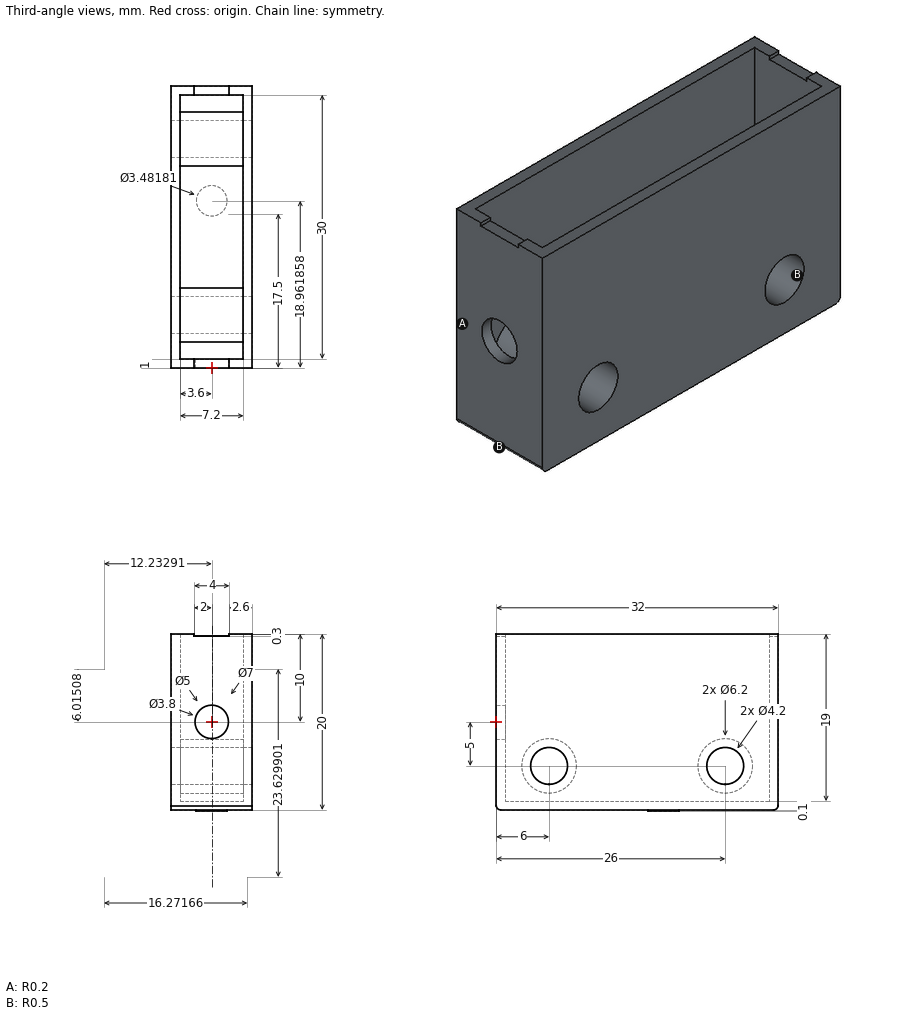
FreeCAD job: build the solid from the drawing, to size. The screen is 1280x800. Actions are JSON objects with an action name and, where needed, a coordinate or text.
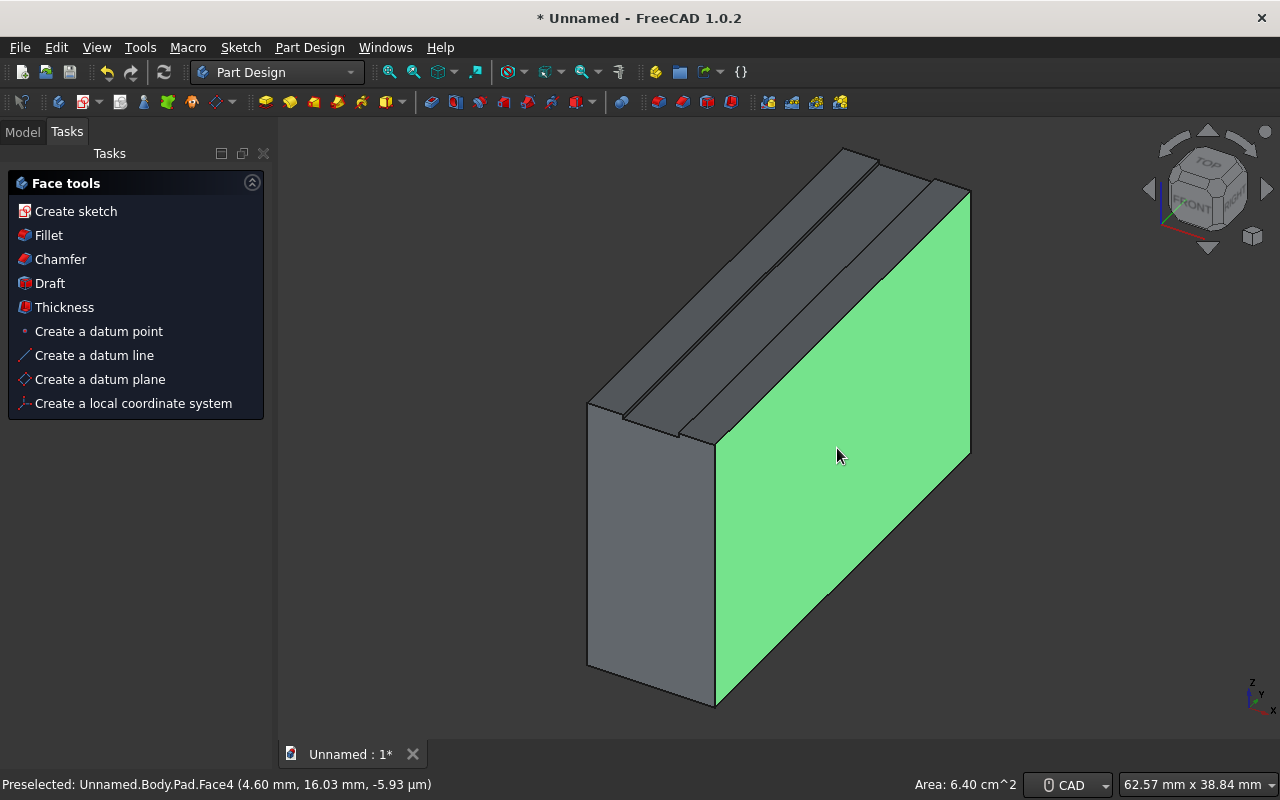
{"action": "left_click", "coordinate": [84, 102]}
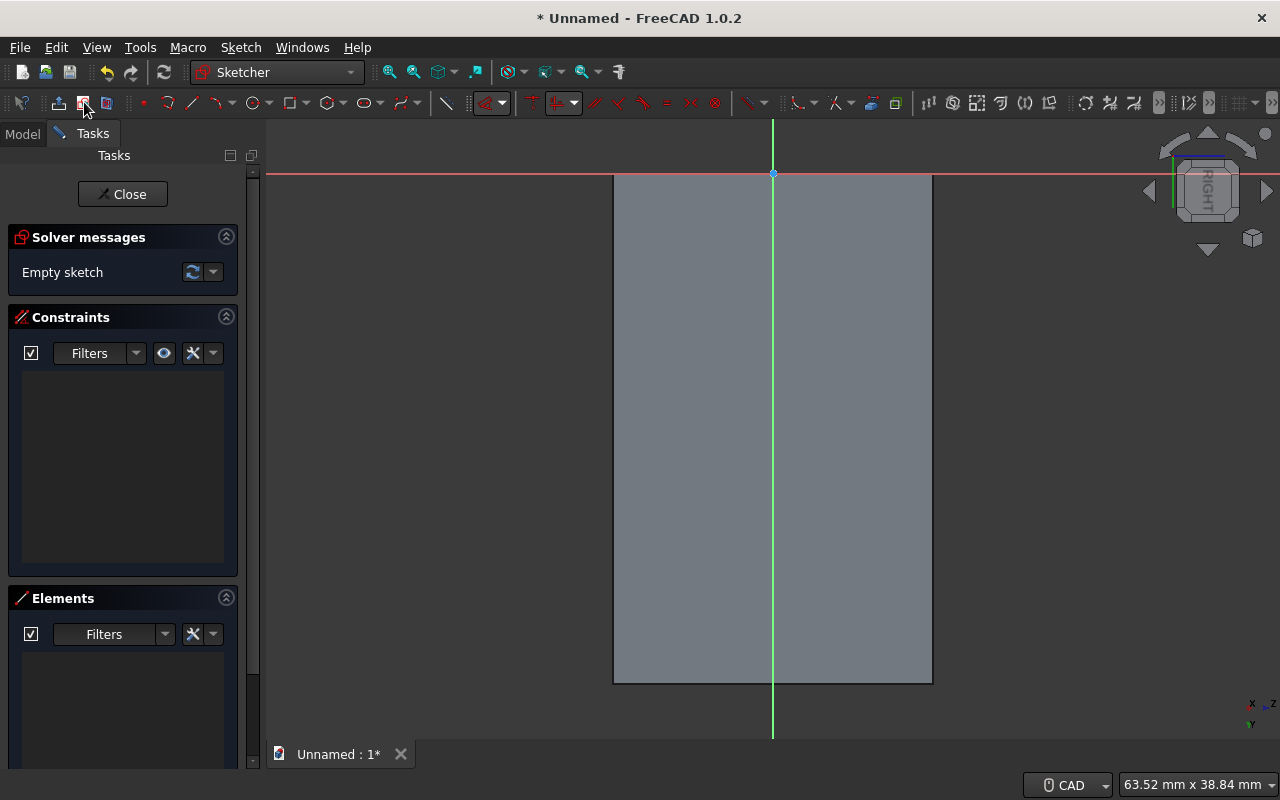
{"action": "left_click", "coordinate": [254, 104]}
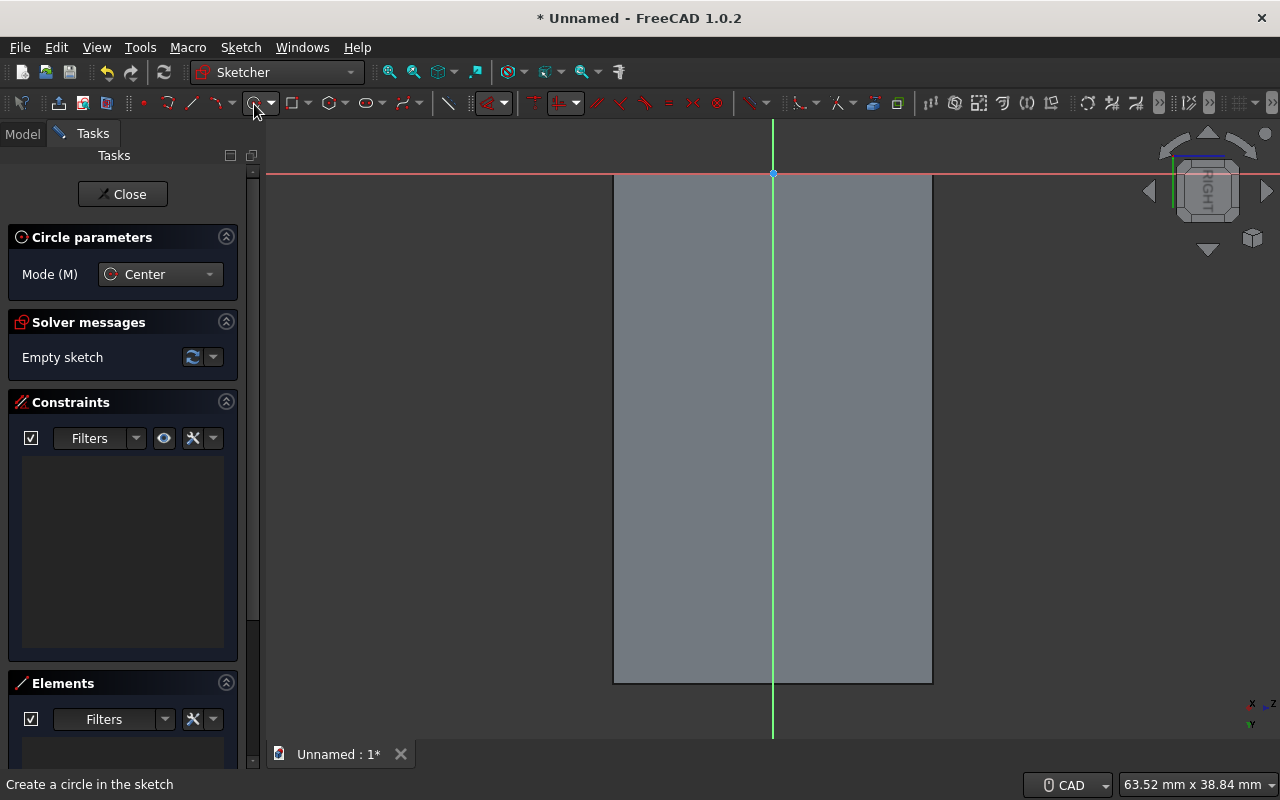
{"action": "left_click", "coordinate": [693, 589]}
{"action": "mouse_move", "coordinate": [717, 565]}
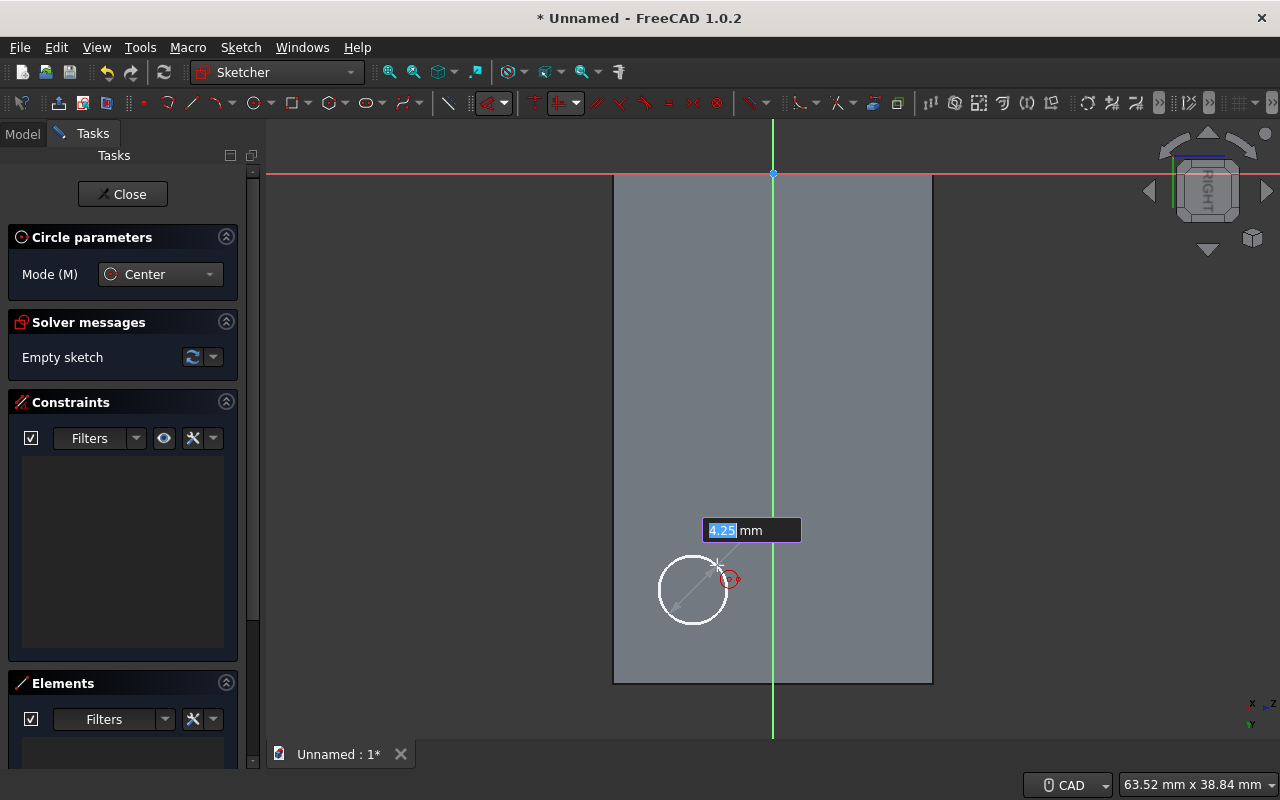
{"action": "type", "text": "4.2"}
{"action": "key", "text": "Return"}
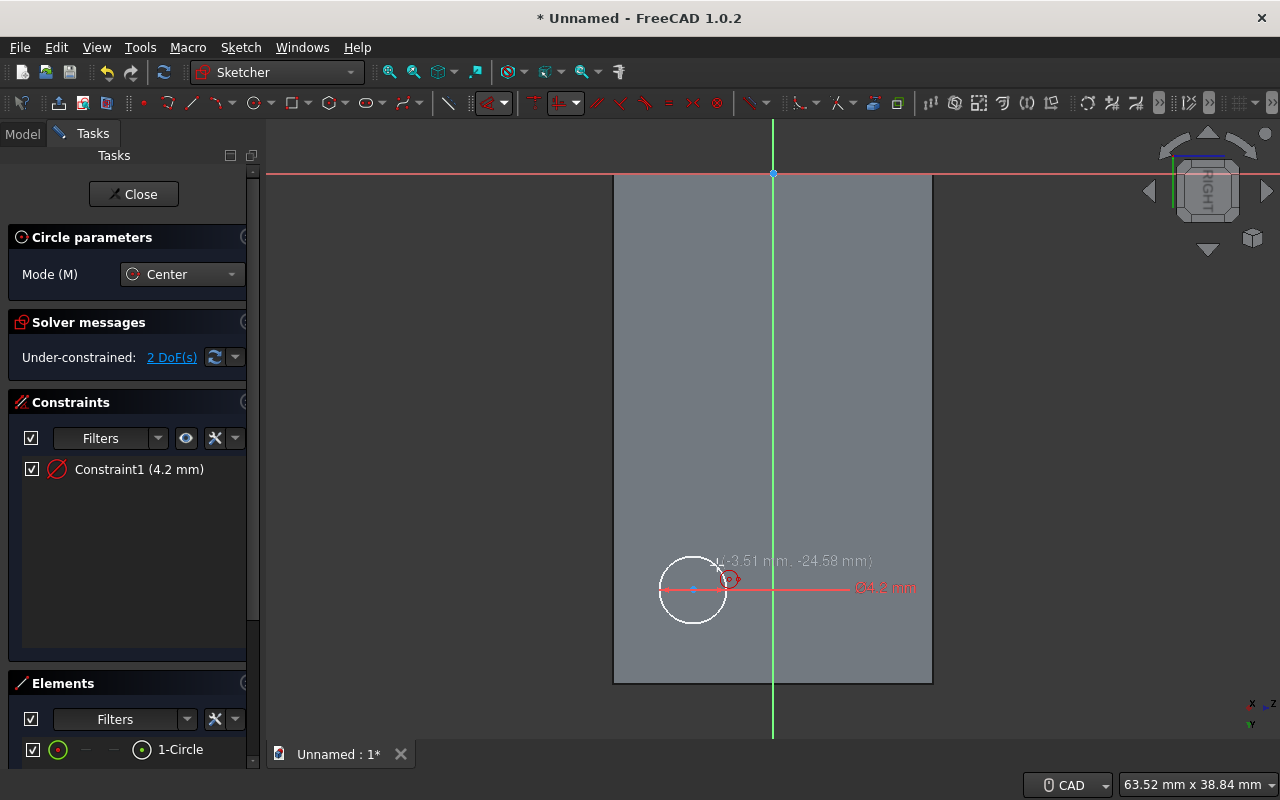
{"action": "left_click", "coordinate": [693, 269]}
{"action": "mouse_move", "coordinate": [717, 246]}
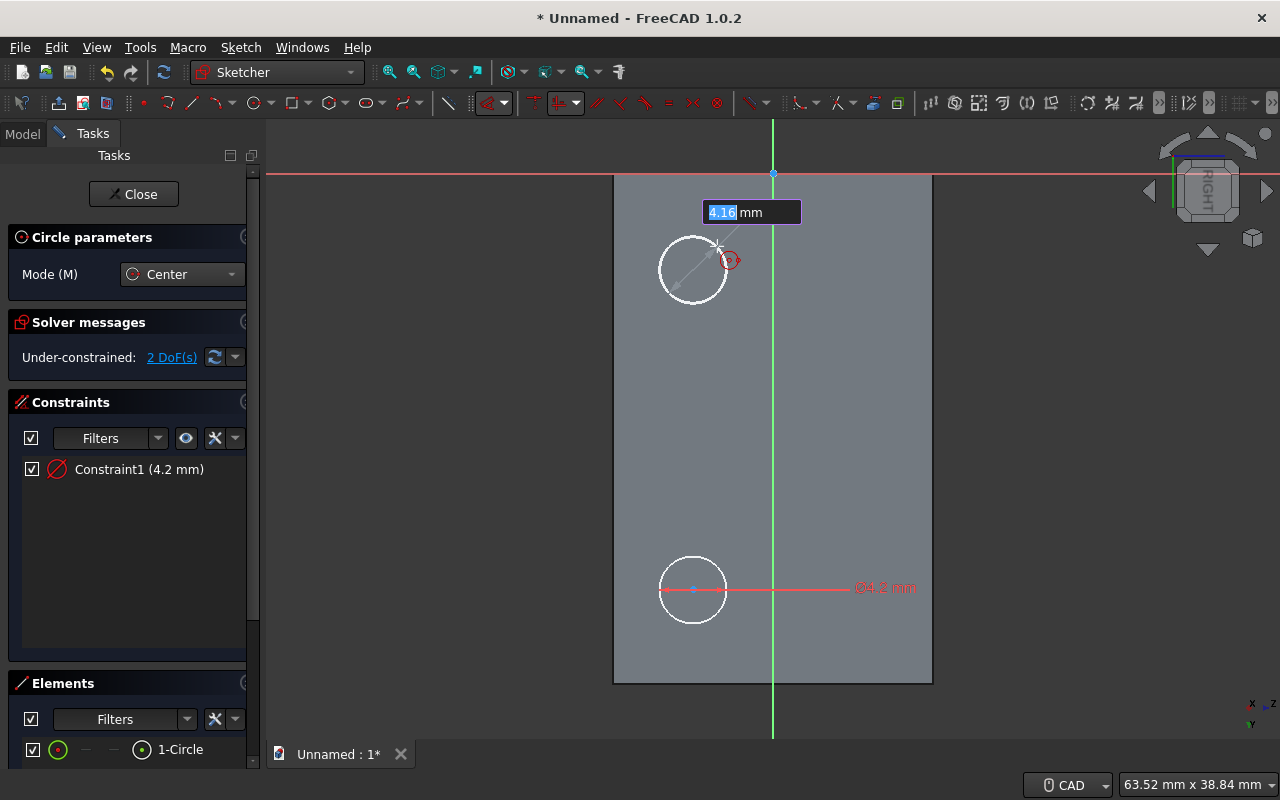
{"action": "type", "text": "4.2"}
{"action": "key", "text": "Return"}
{"action": "key", "text": "Escape"}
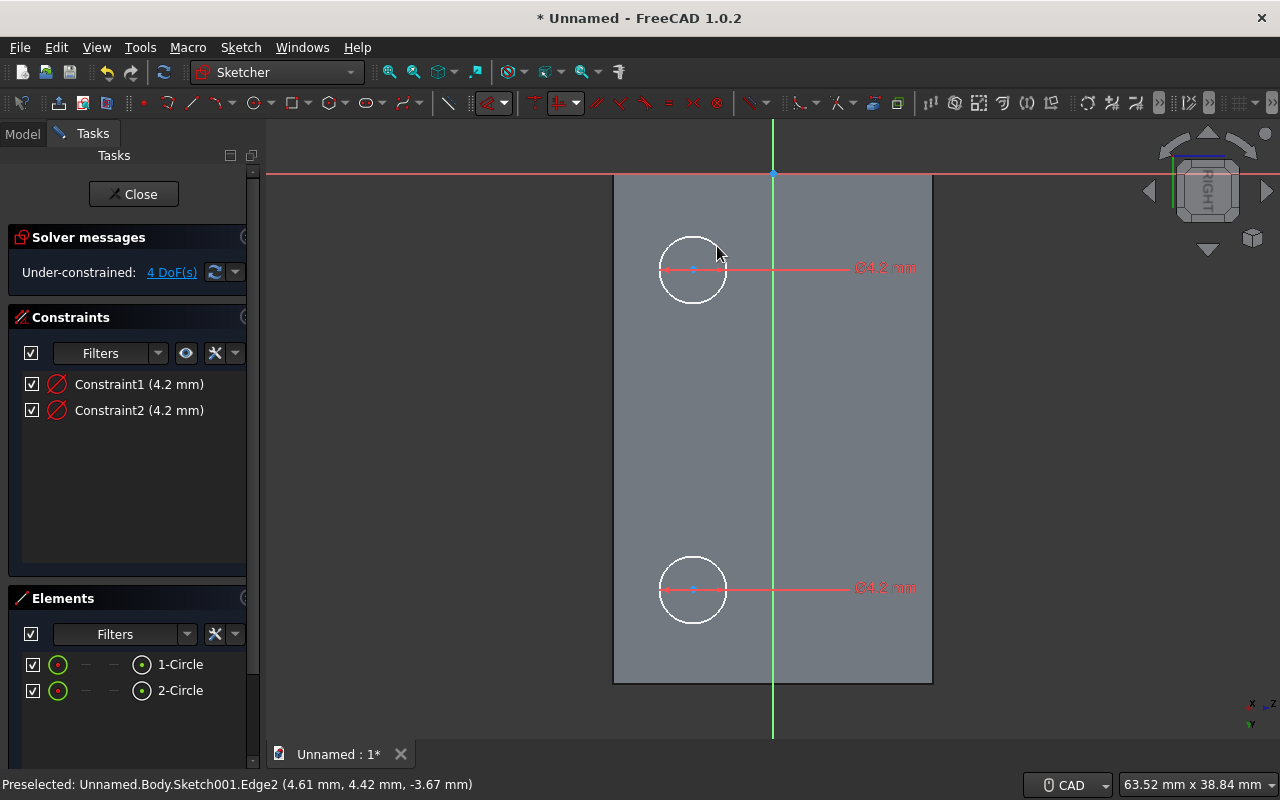
{"action": "left_click", "coordinate": [693, 590]}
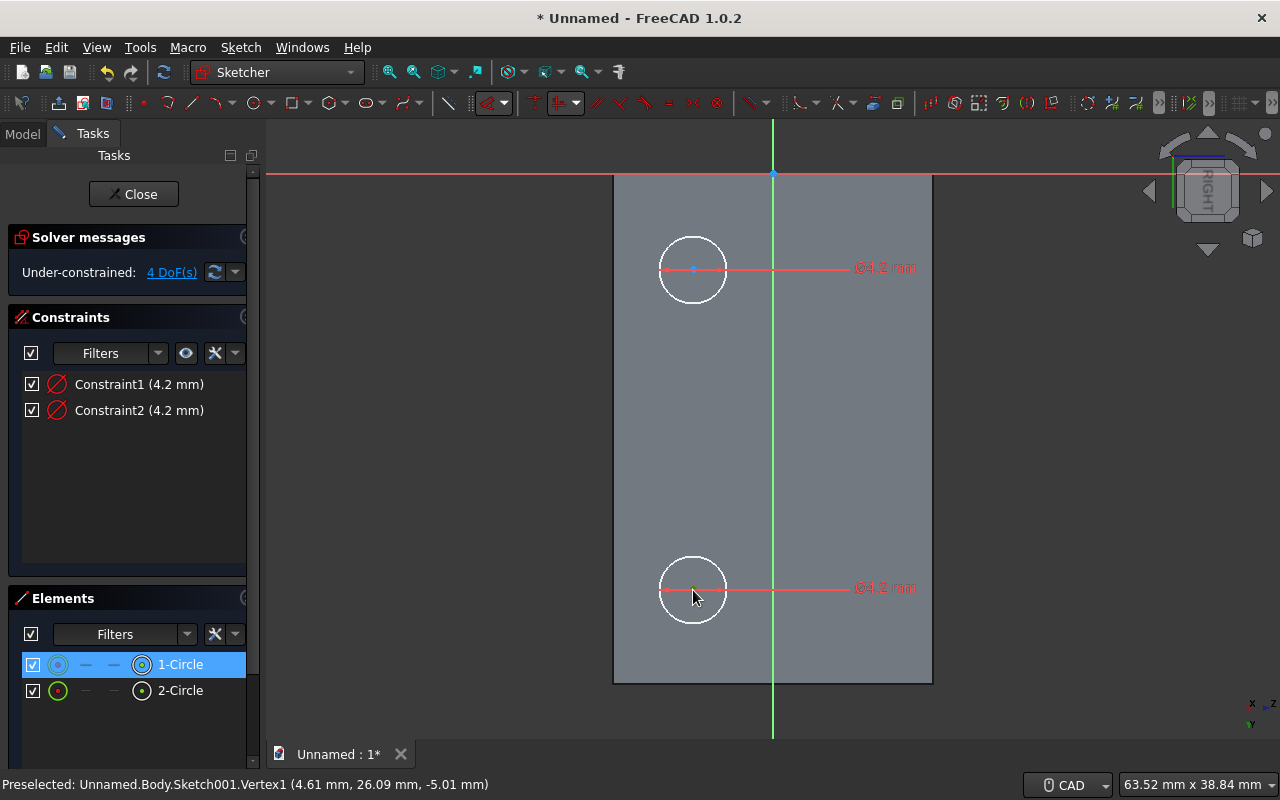
{"action": "left_click", "coordinate": [693, 270]}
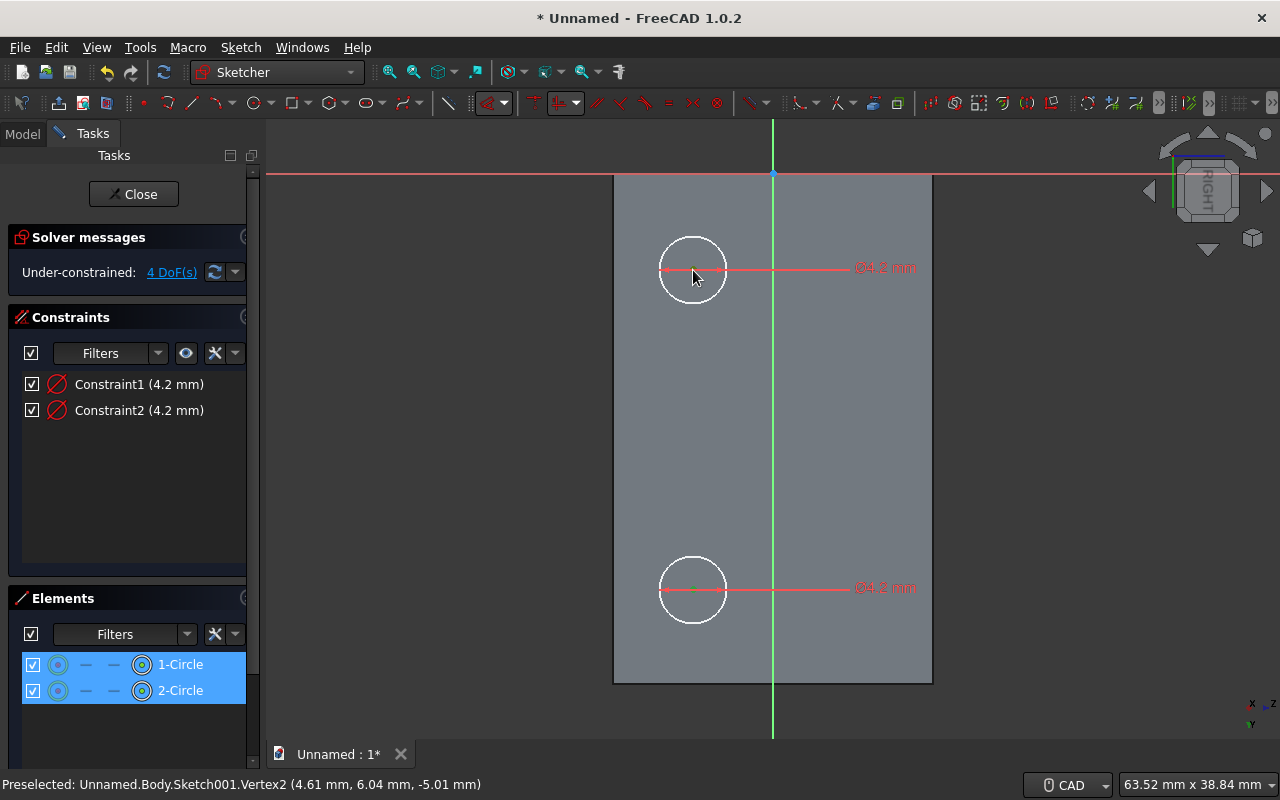
{"action": "key", "text": "v"}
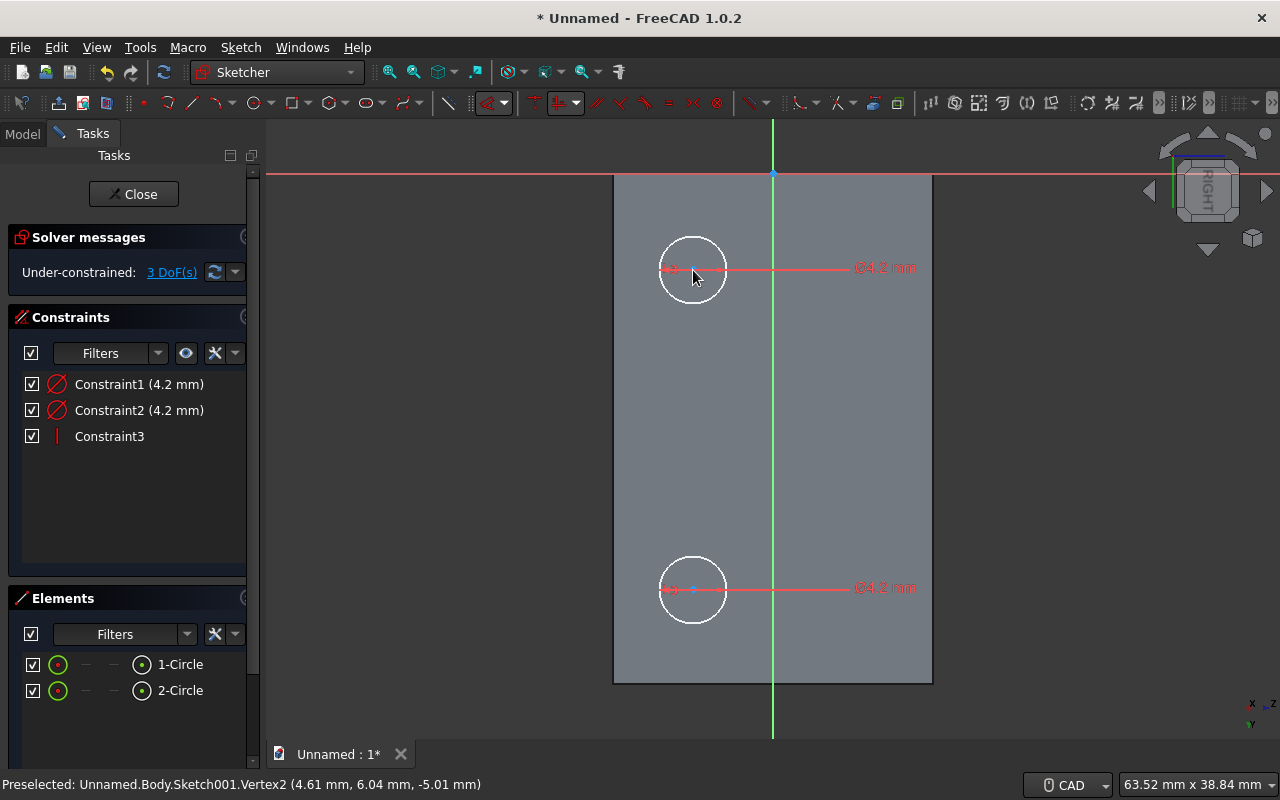
{"action": "left_click", "coordinate": [693, 590]}